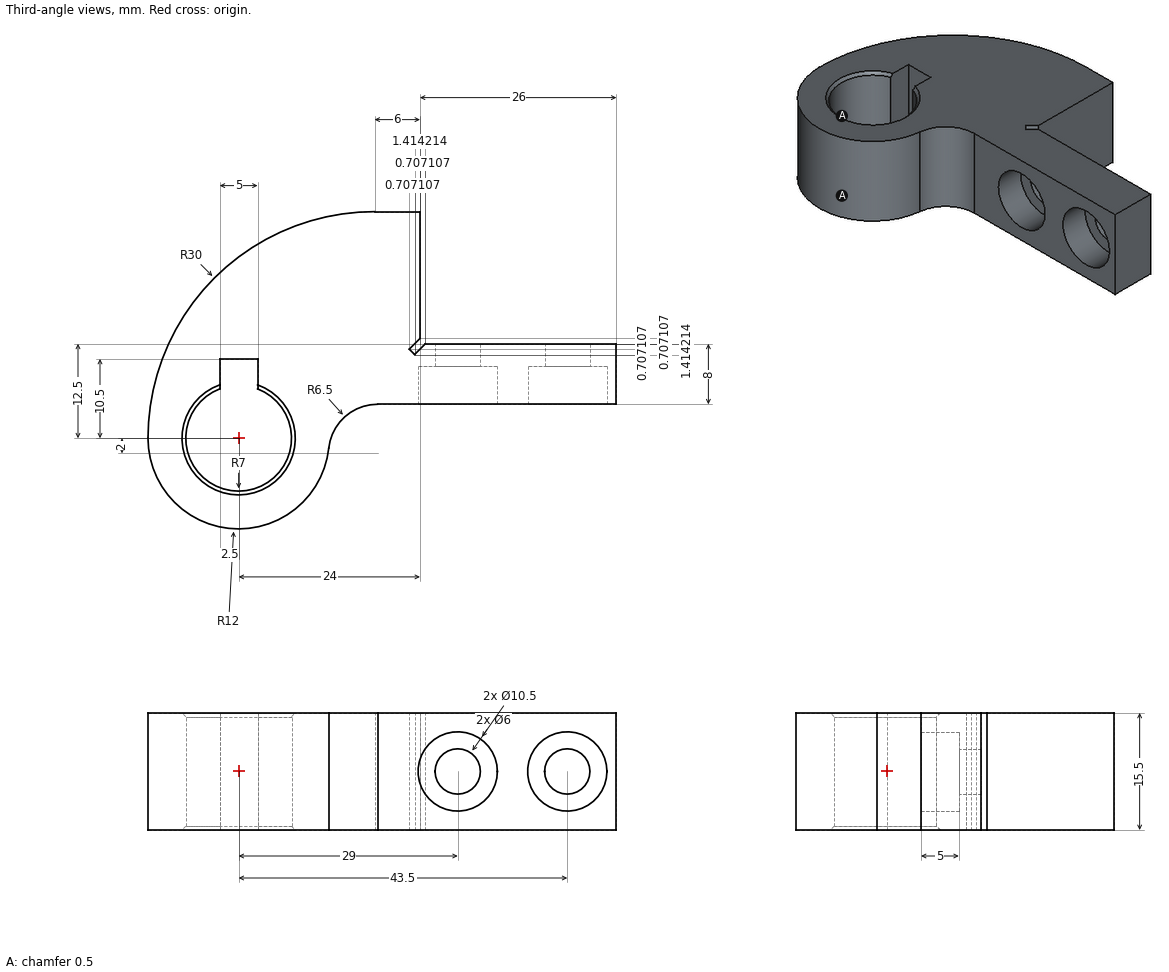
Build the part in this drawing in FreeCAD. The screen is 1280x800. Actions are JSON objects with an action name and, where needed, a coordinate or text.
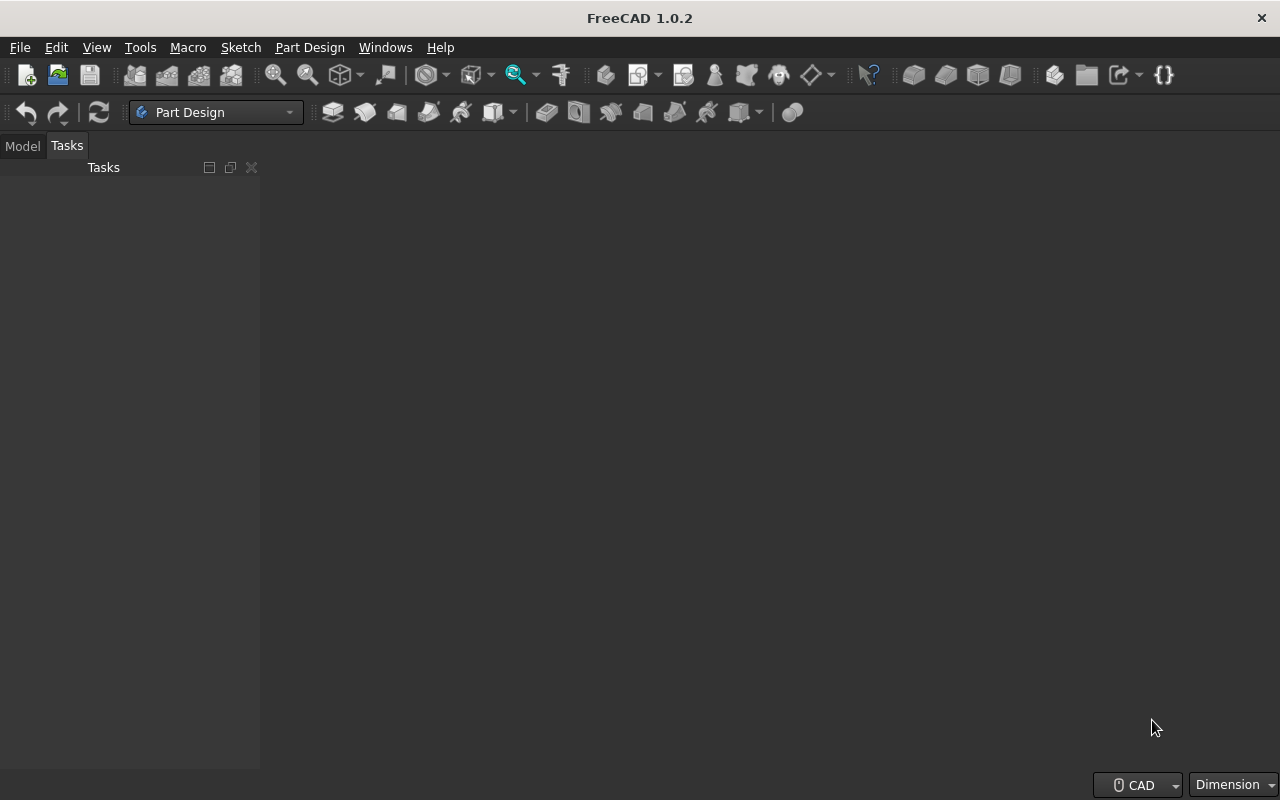
{"action": "left_click", "coordinate": [26, 76]}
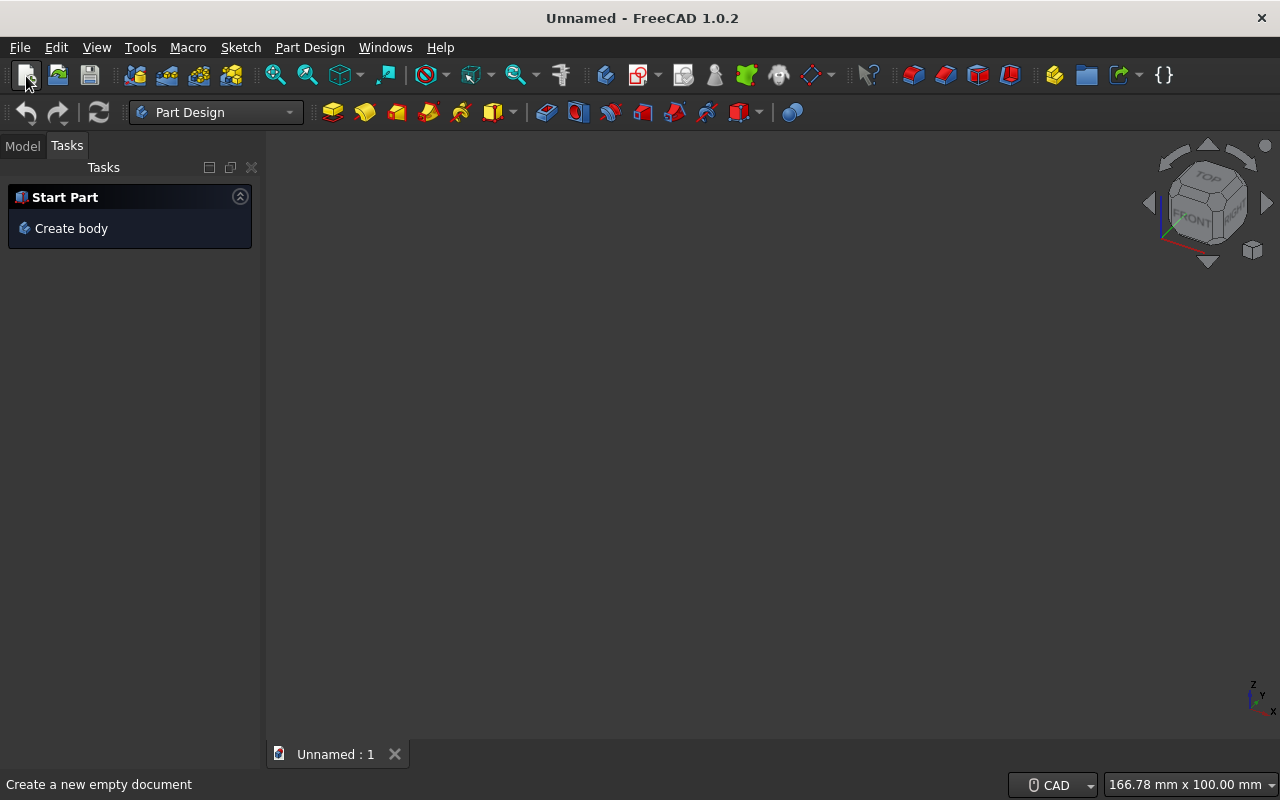
{"action": "left_click", "coordinate": [638, 76]}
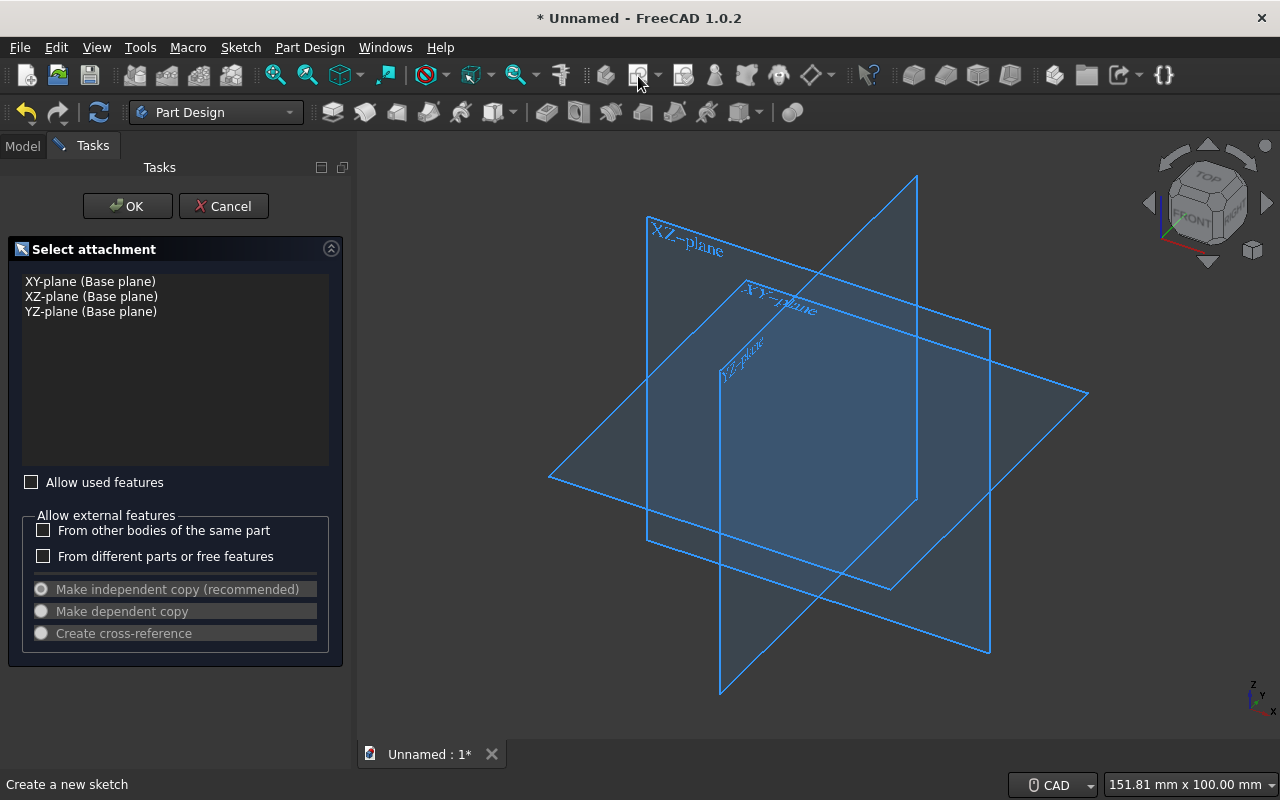
{"action": "left_click", "coordinate": [82, 282]}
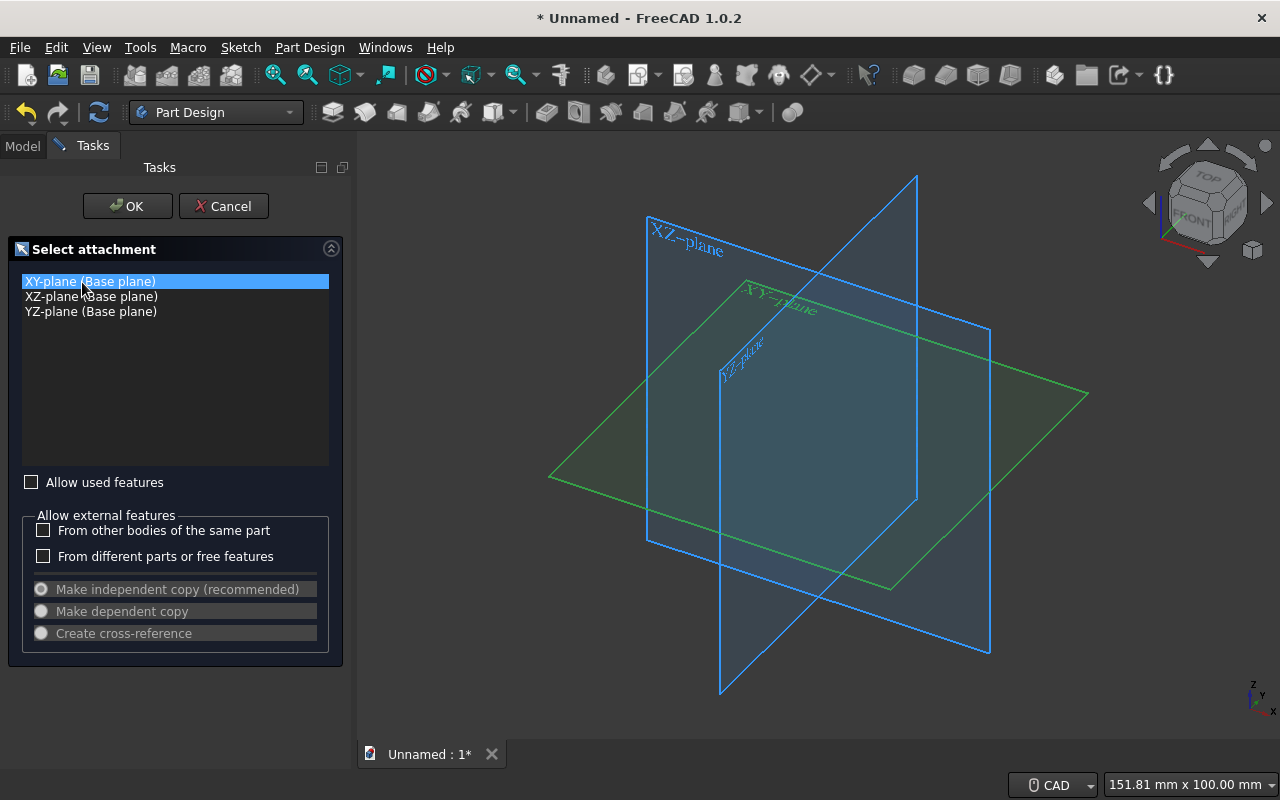
{"action": "left_click", "coordinate": [128, 206]}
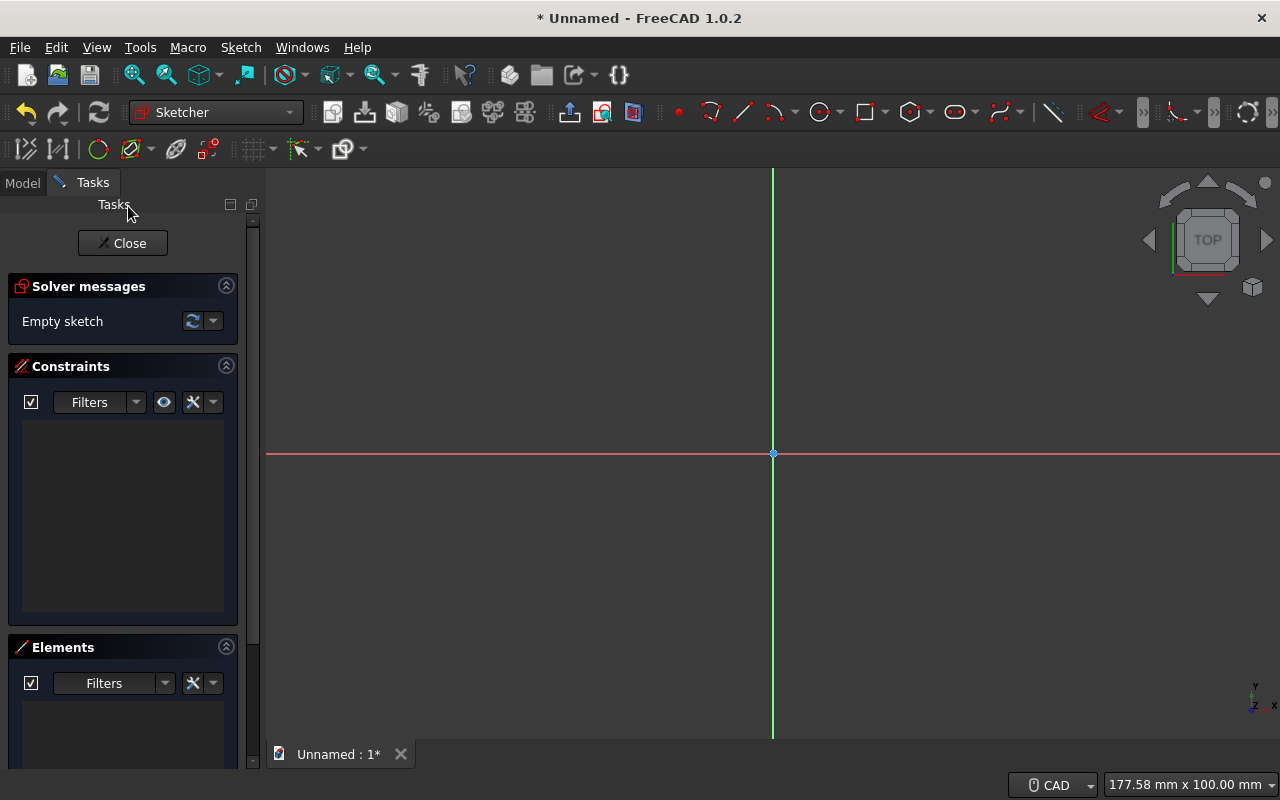
{"action": "scroll", "coordinate": [1115, 297], "scroll_direction": "up", "scroll_amount": 2}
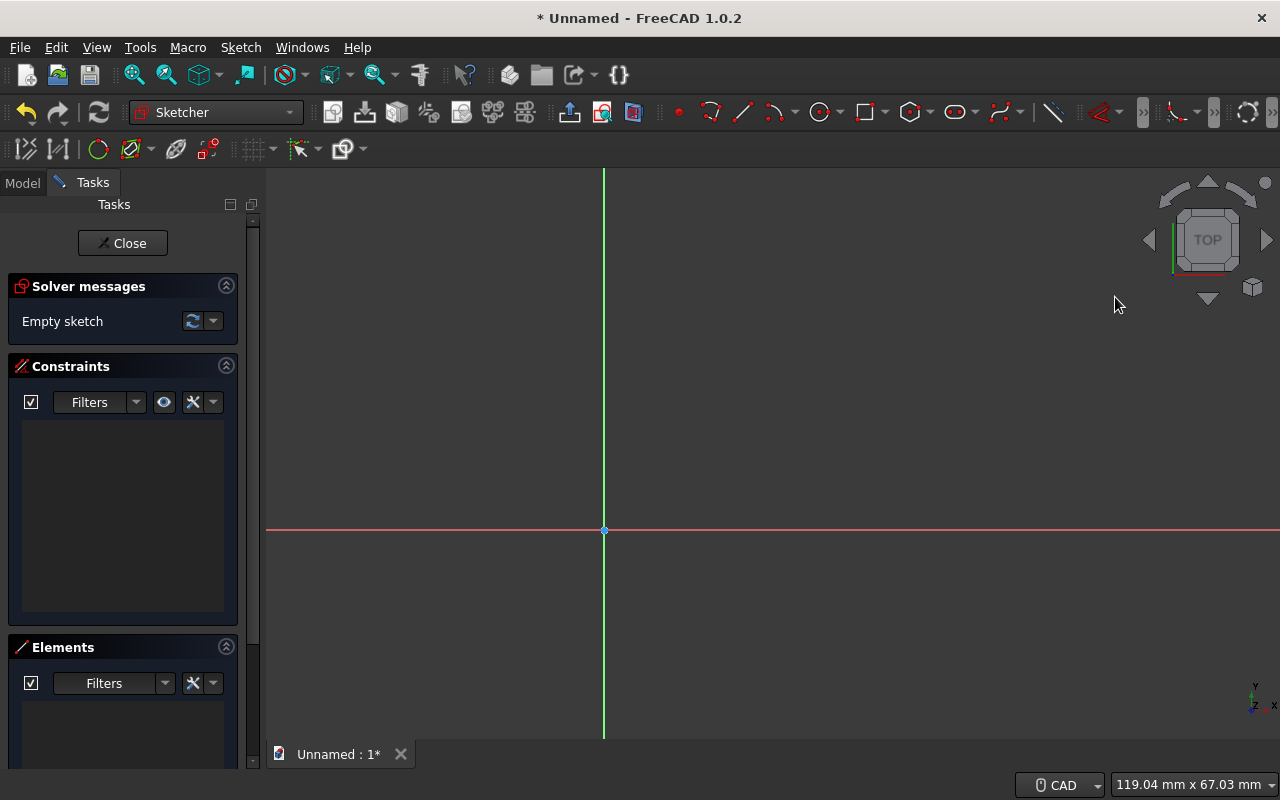
{"action": "left_click", "coordinate": [712, 112]}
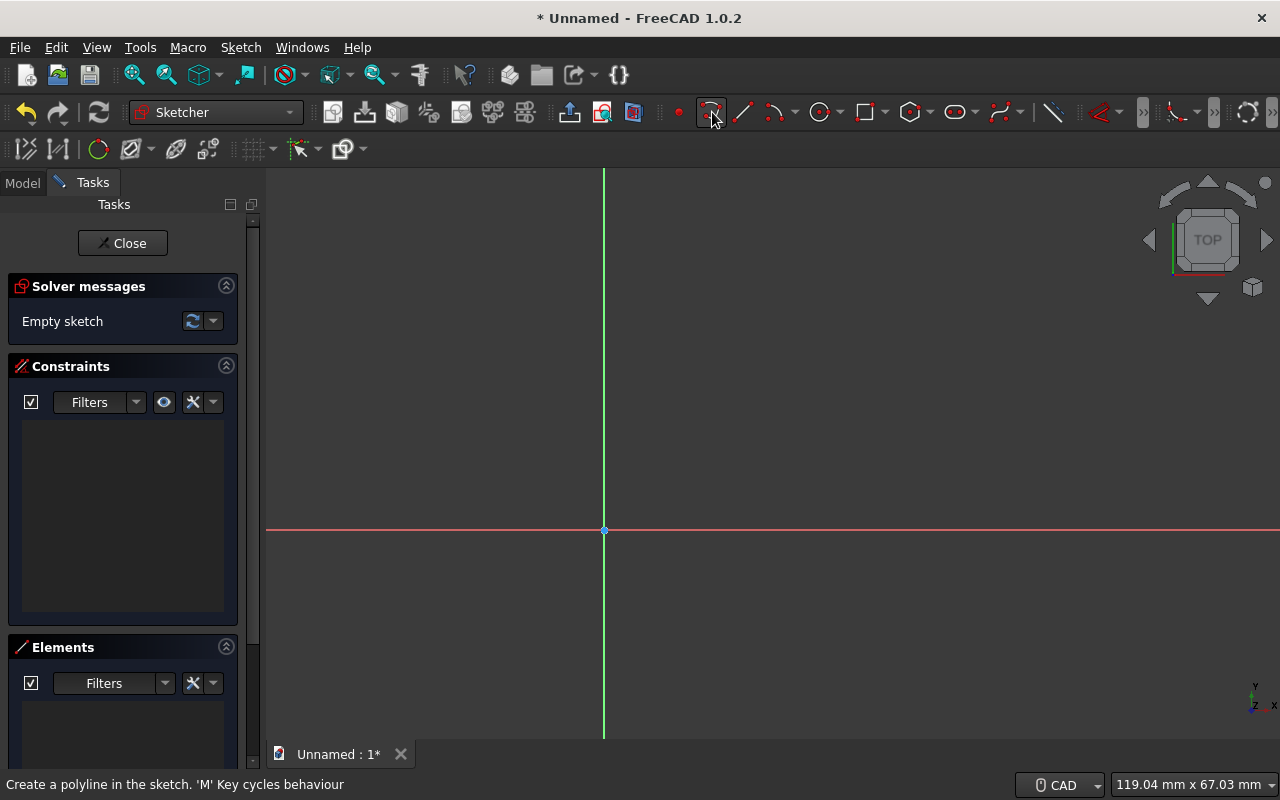
{"action": "left_click", "coordinate": [761, 492]}
{"action": "left_click", "coordinate": [1030, 492]}
{"action": "left_click", "coordinate": [1030, 424]}
{"action": "left_click", "coordinate": [809, 424]}
{"action": "left_click", "coordinate": [809, 275]}
{"action": "left_click", "coordinate": [758, 275]}
{"action": "right_click", "coordinate": [758, 275]}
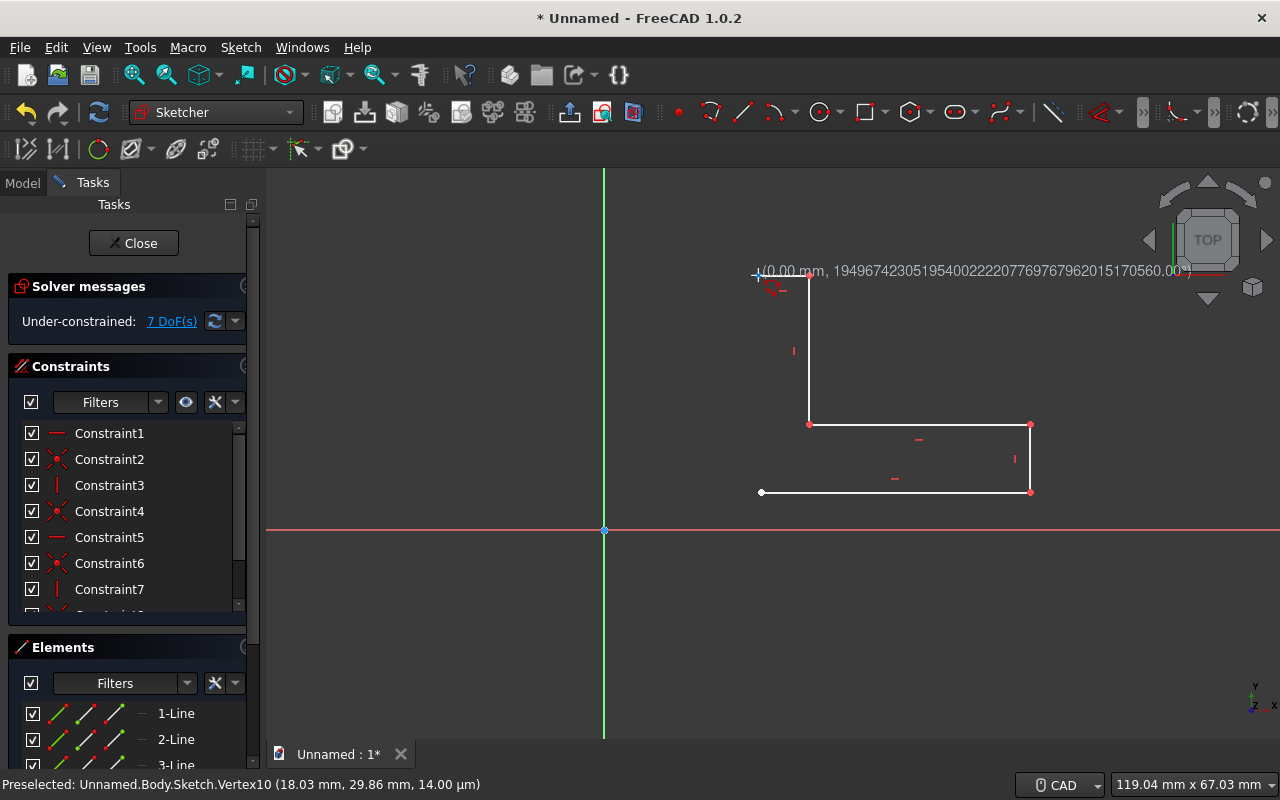
{"action": "left_click", "coordinate": [798, 112]}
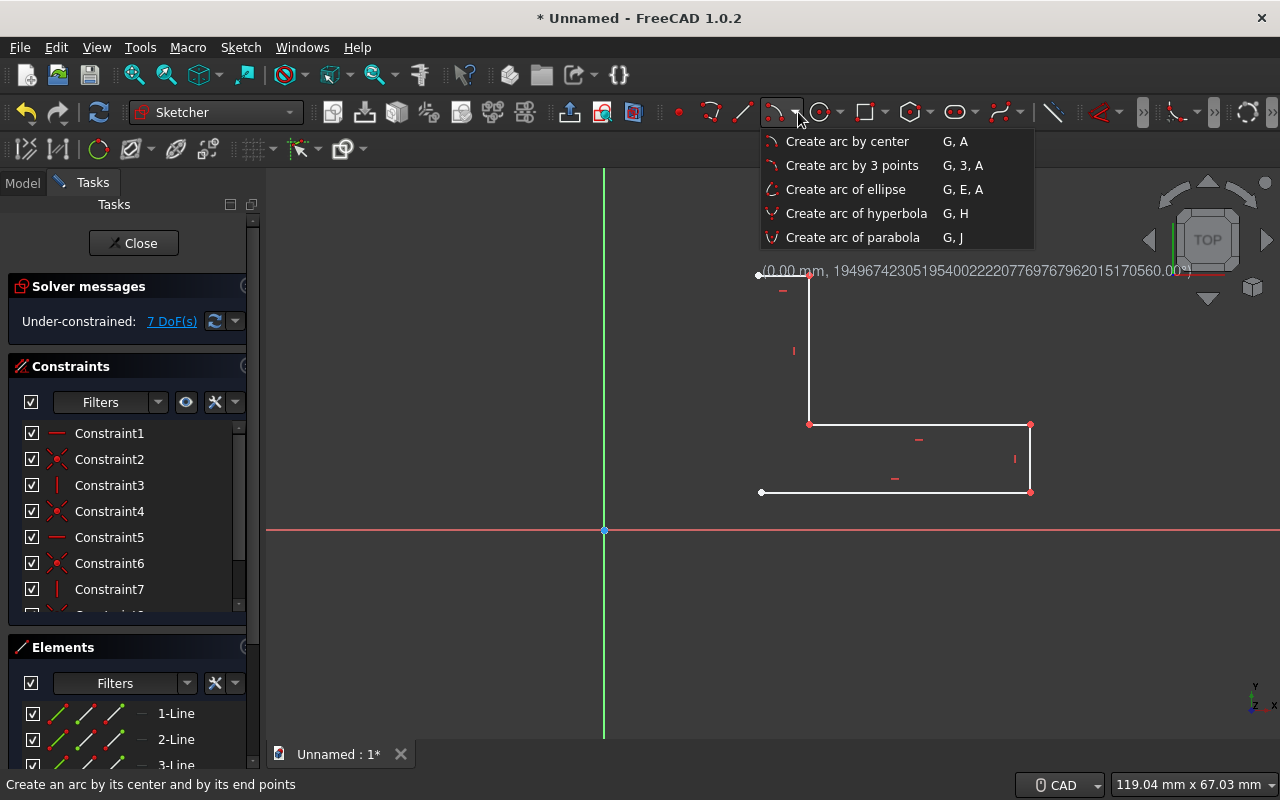
{"action": "left_click", "coordinate": [898, 165]}